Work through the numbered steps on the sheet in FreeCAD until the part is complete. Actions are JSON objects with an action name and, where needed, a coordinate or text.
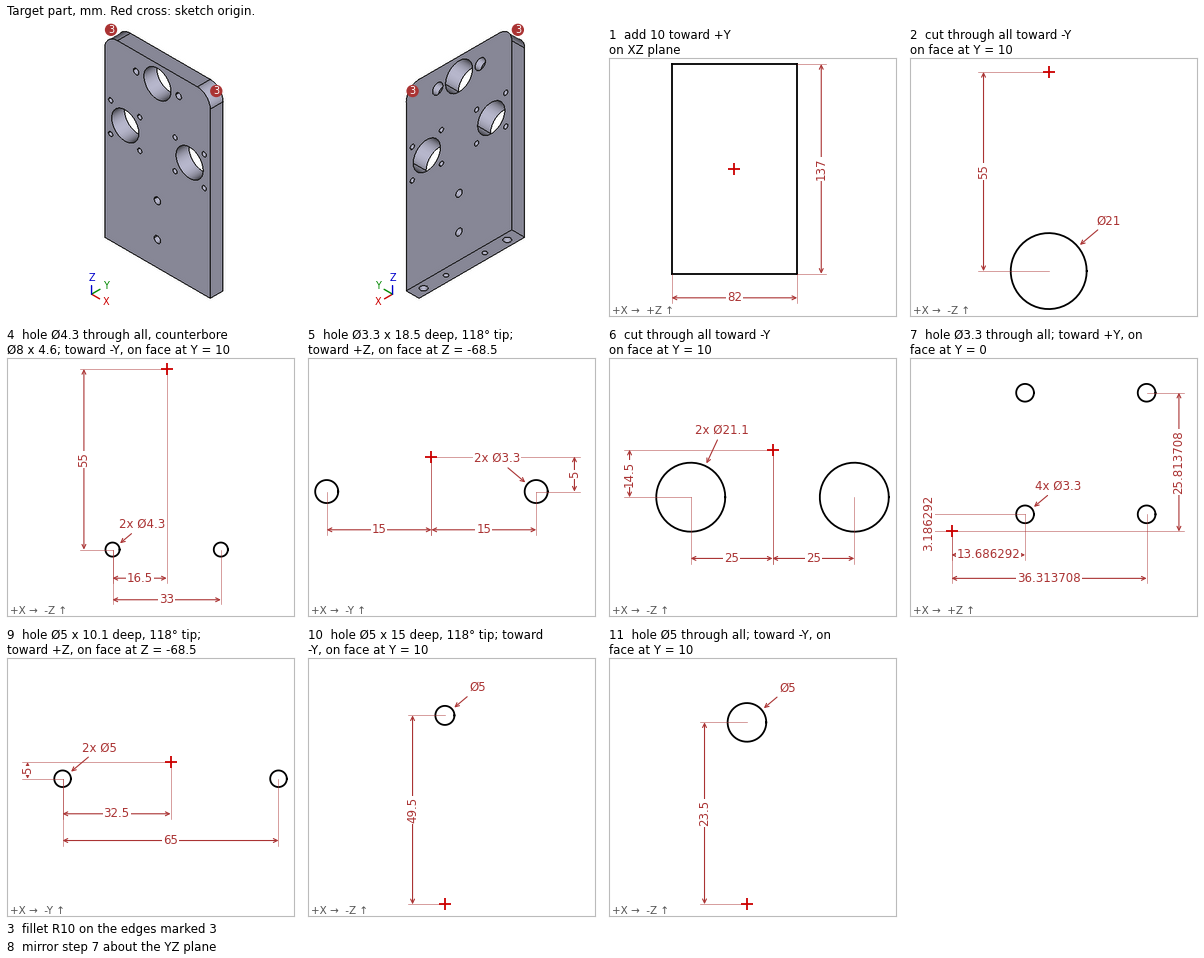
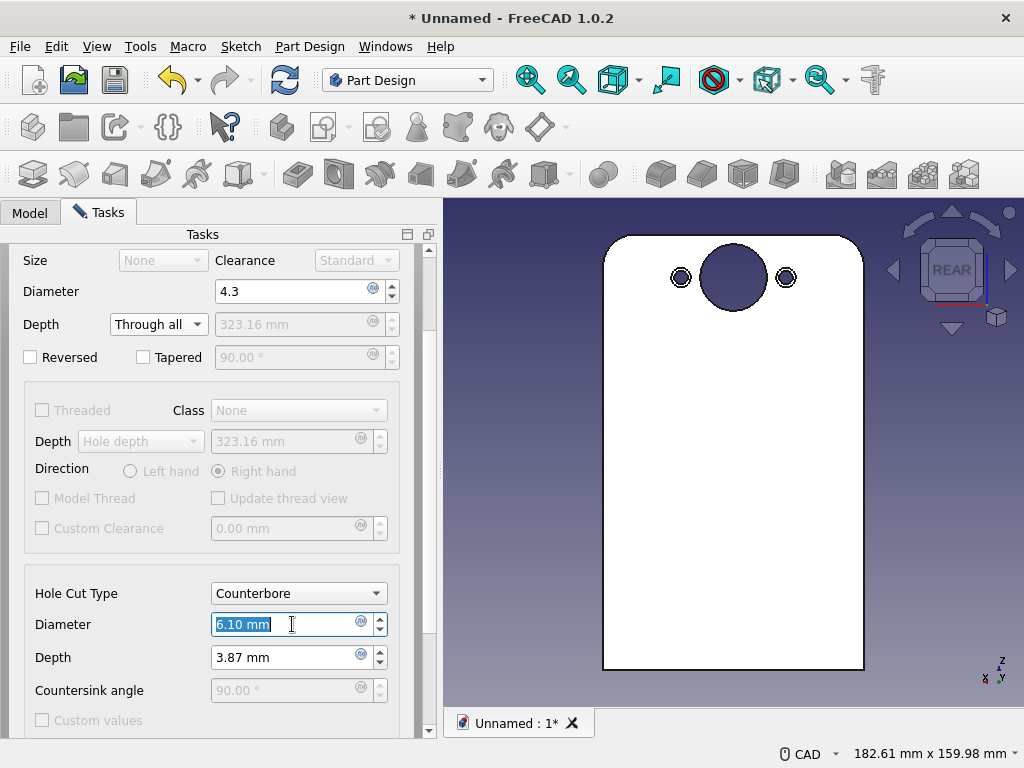
{"action": "type", "text": "8"}
{"action": "key", "text": "Tab"}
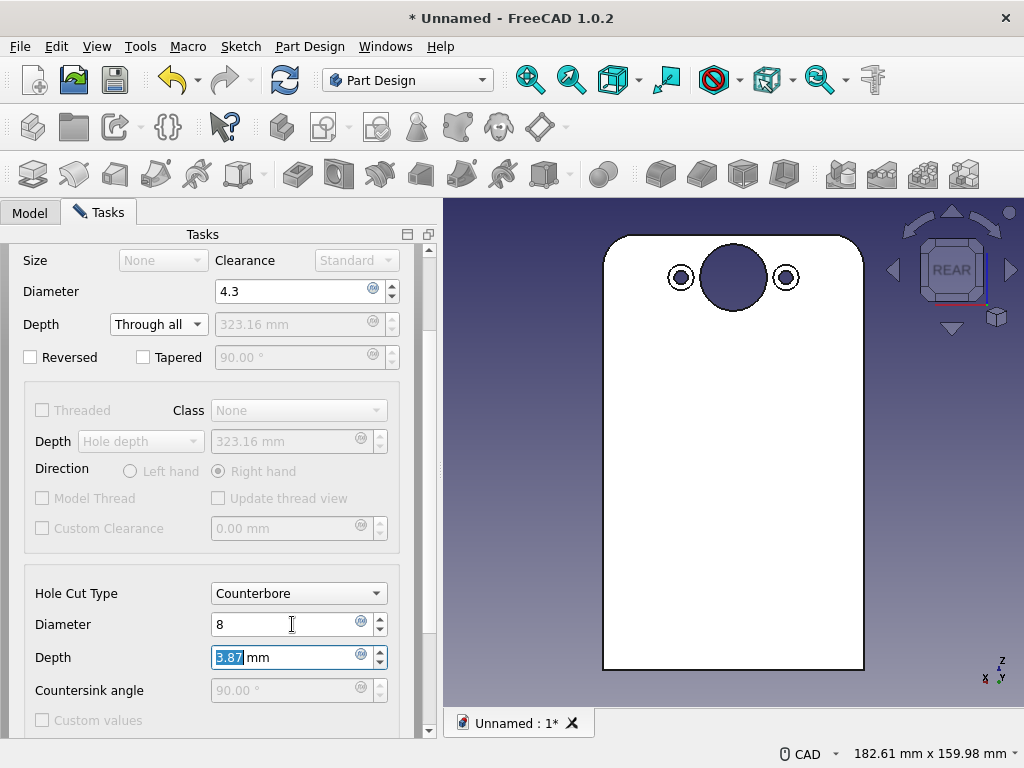
{"action": "type", "text": "4.6"}
{"action": "key", "text": "Tab"}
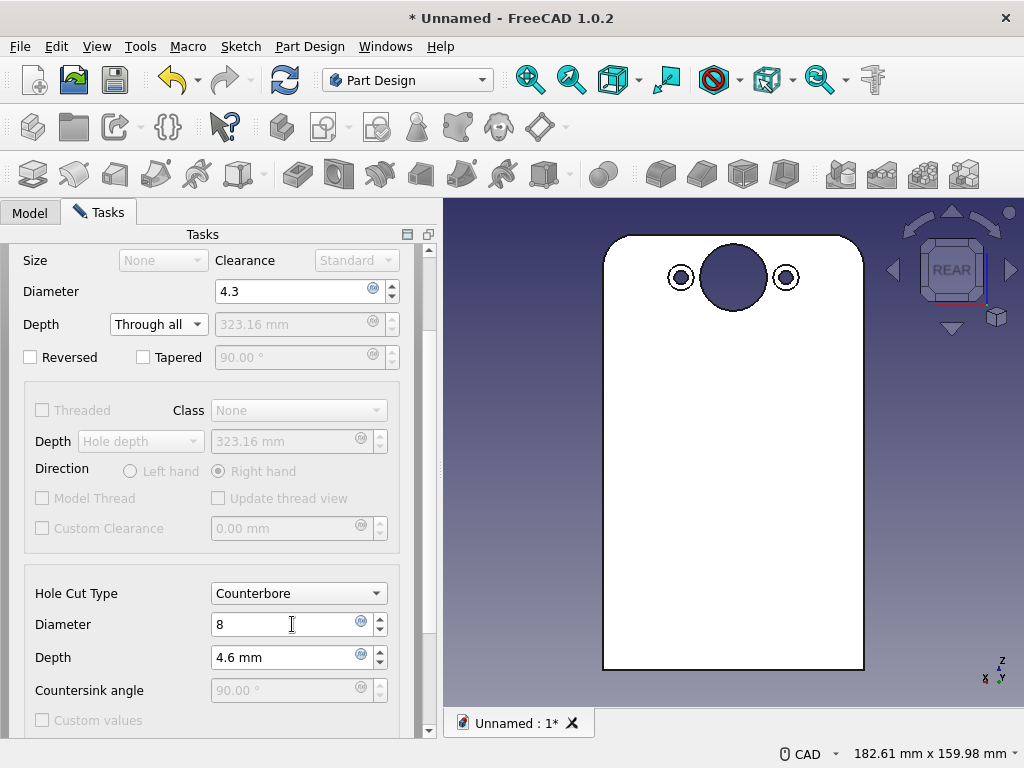
{"action": "scroll", "coordinate": [429, 491], "scroll_direction": "up", "scroll_amount": 3}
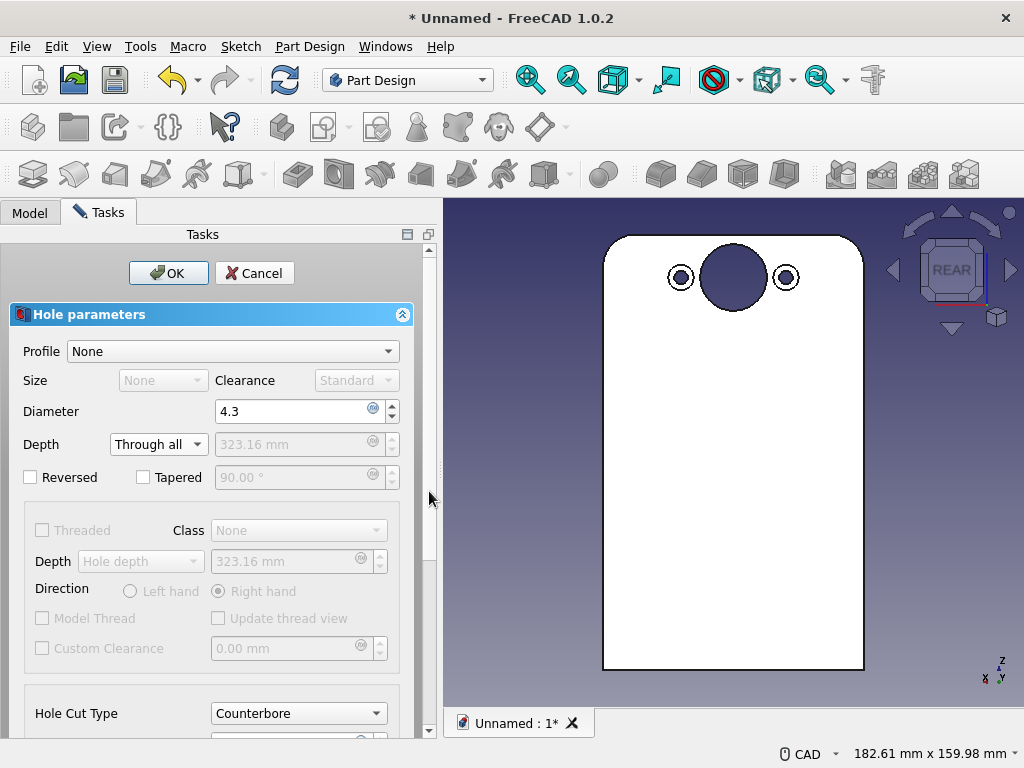
{"action": "left_click", "coordinate": [169, 273]}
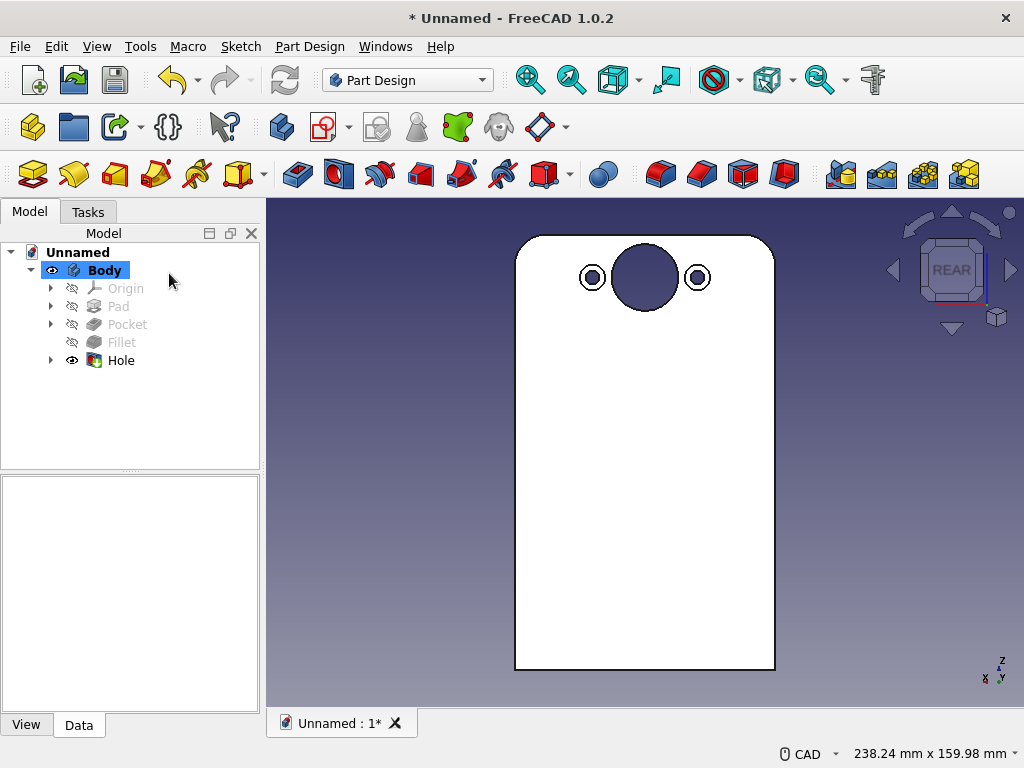
{"action": "key", "text": "5"}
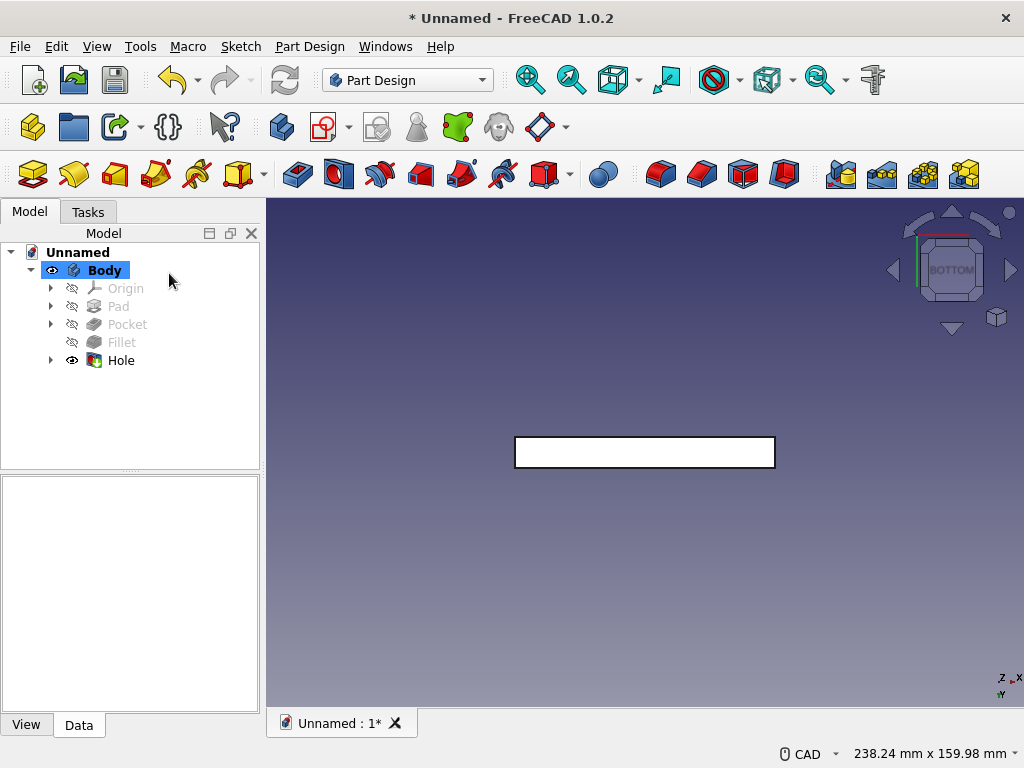
{"action": "key", "text": "v f"}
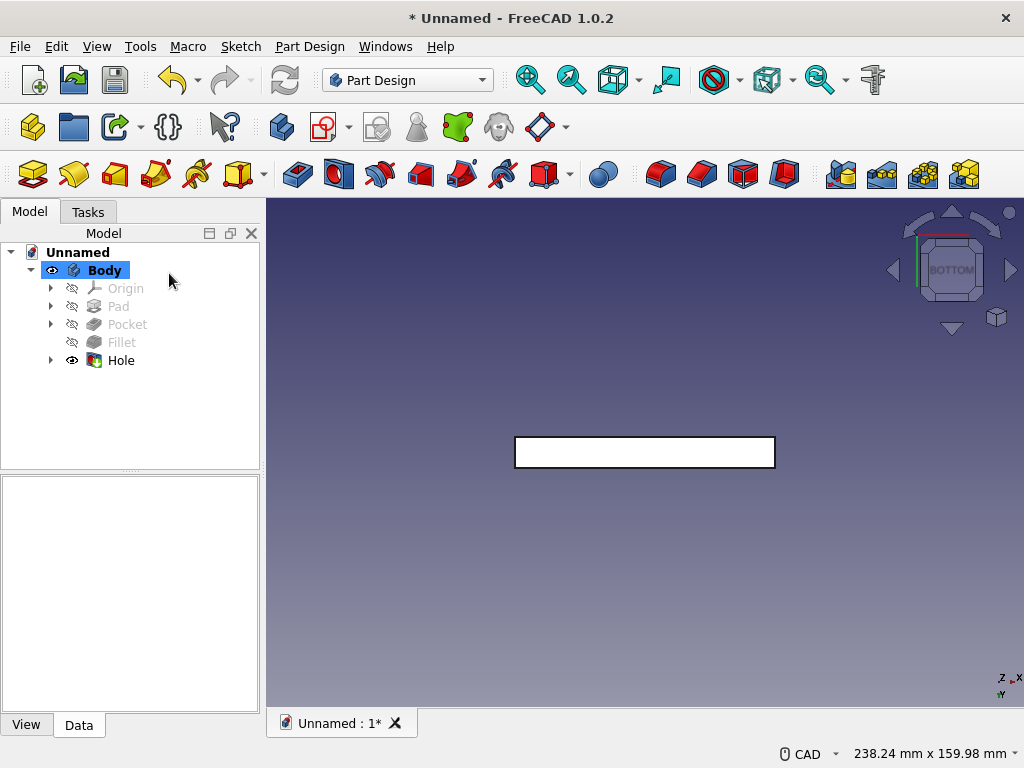
{"action": "left_click", "coordinate": [757, 451]}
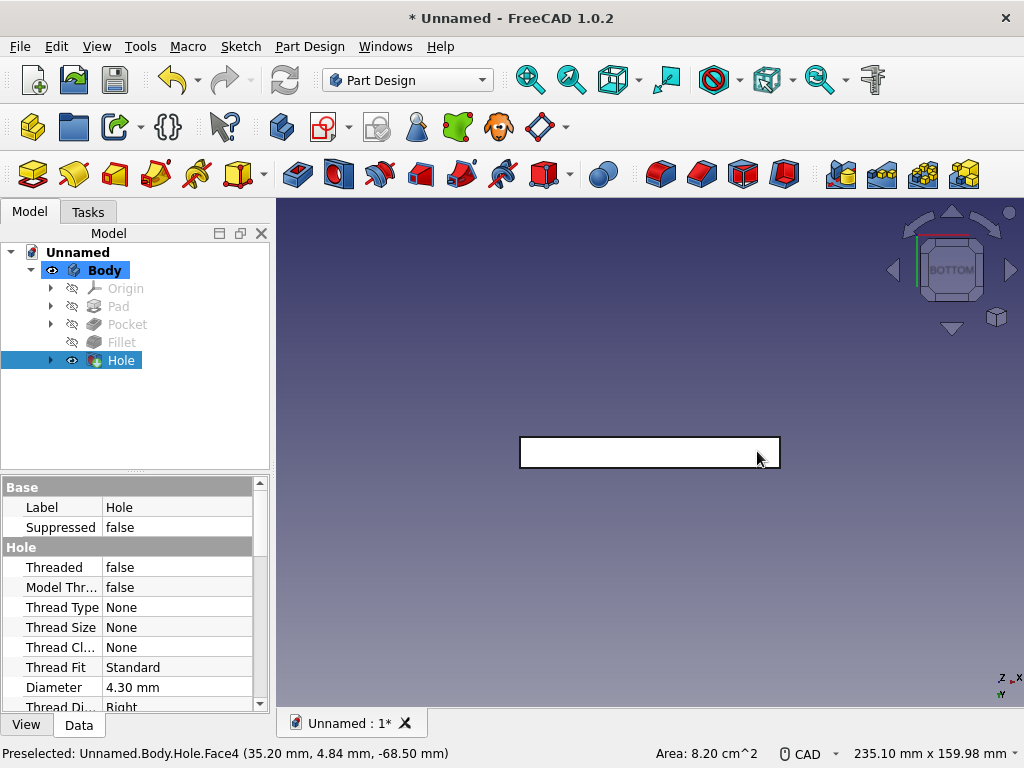
{"action": "left_click", "coordinate": [322, 128]}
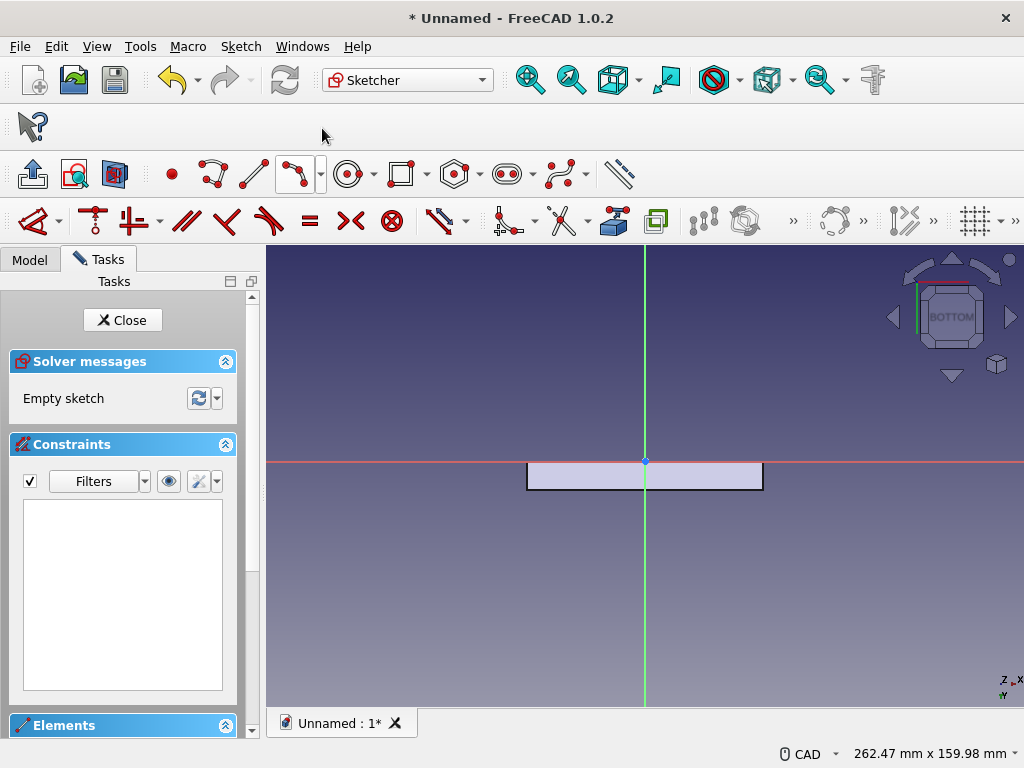
{"action": "scroll", "coordinate": [667, 470], "scroll_direction": "up", "scroll_amount": 7}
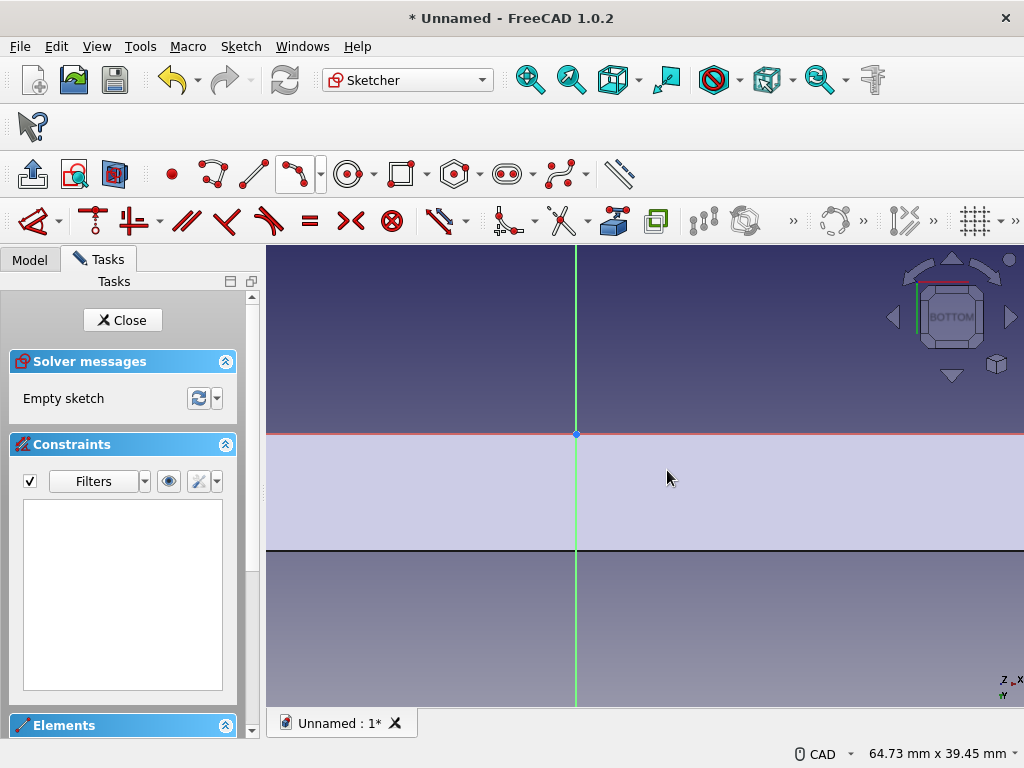
{"action": "left_click", "coordinate": [348, 174]}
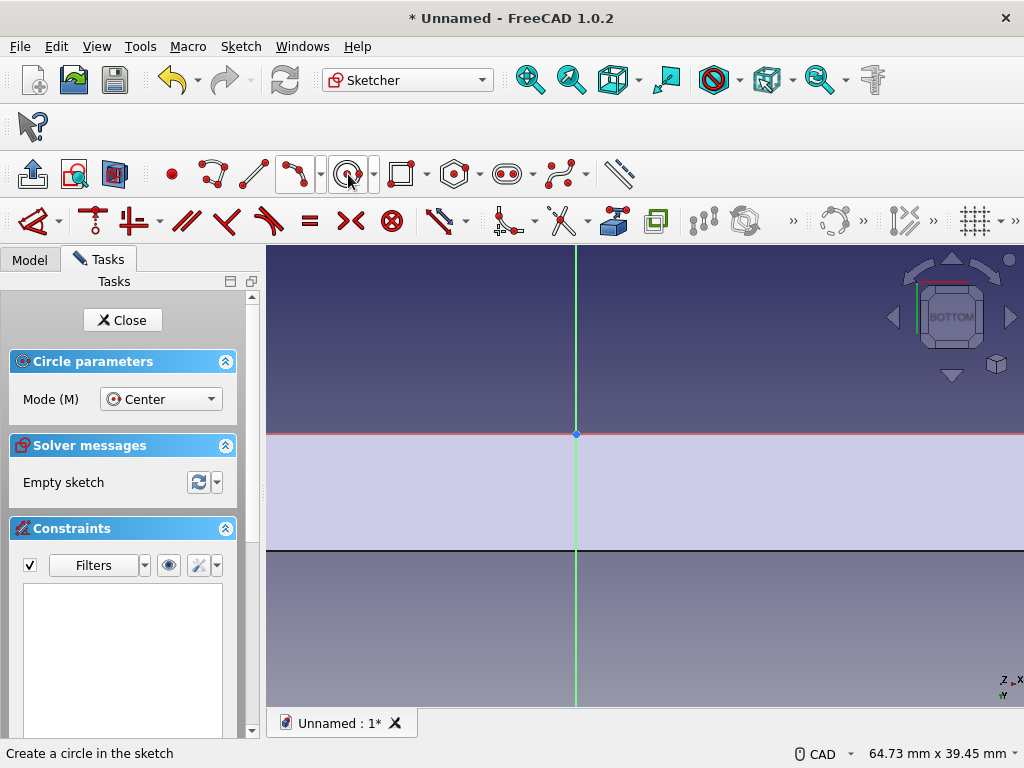
{"action": "left_click", "coordinate": [752, 493]}
{"action": "mouse_move", "coordinate": [765, 479]}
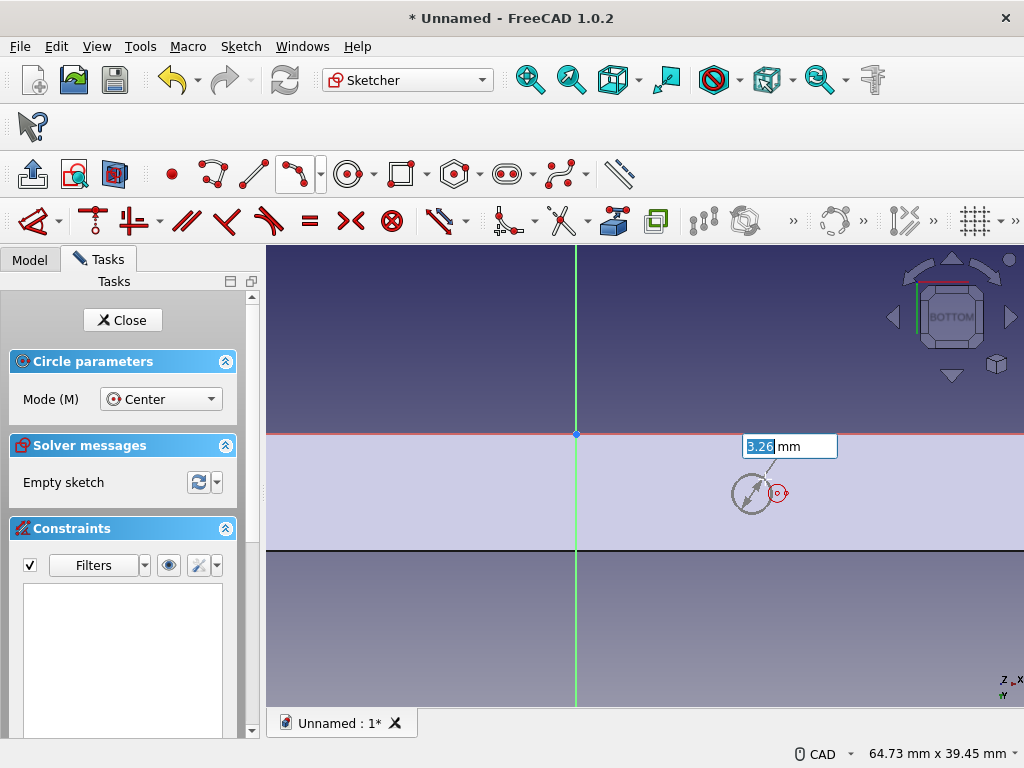
{"action": "type", "text": "3.3"}
{"action": "key", "text": "Return"}